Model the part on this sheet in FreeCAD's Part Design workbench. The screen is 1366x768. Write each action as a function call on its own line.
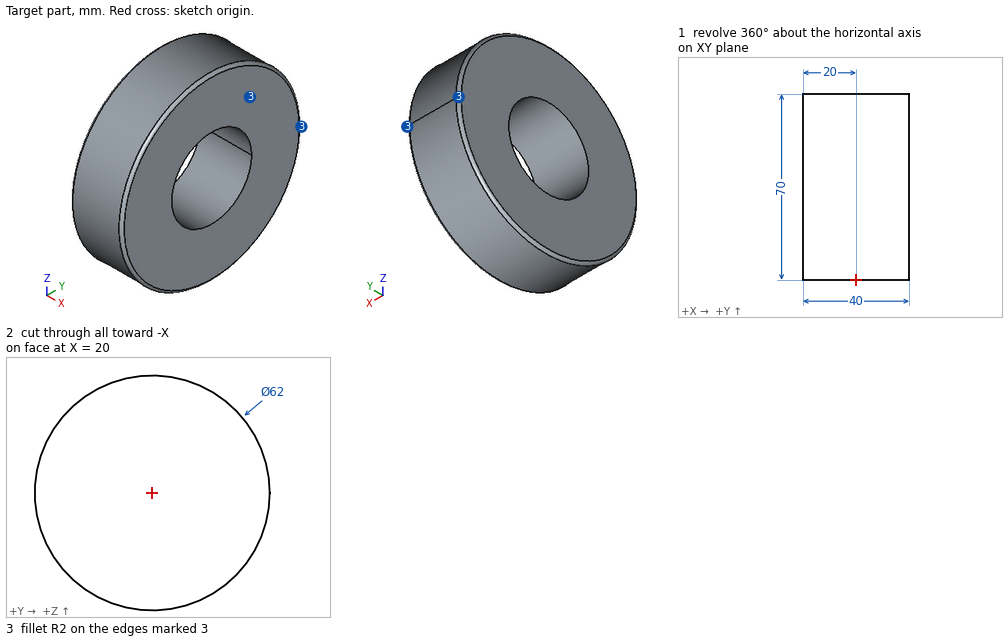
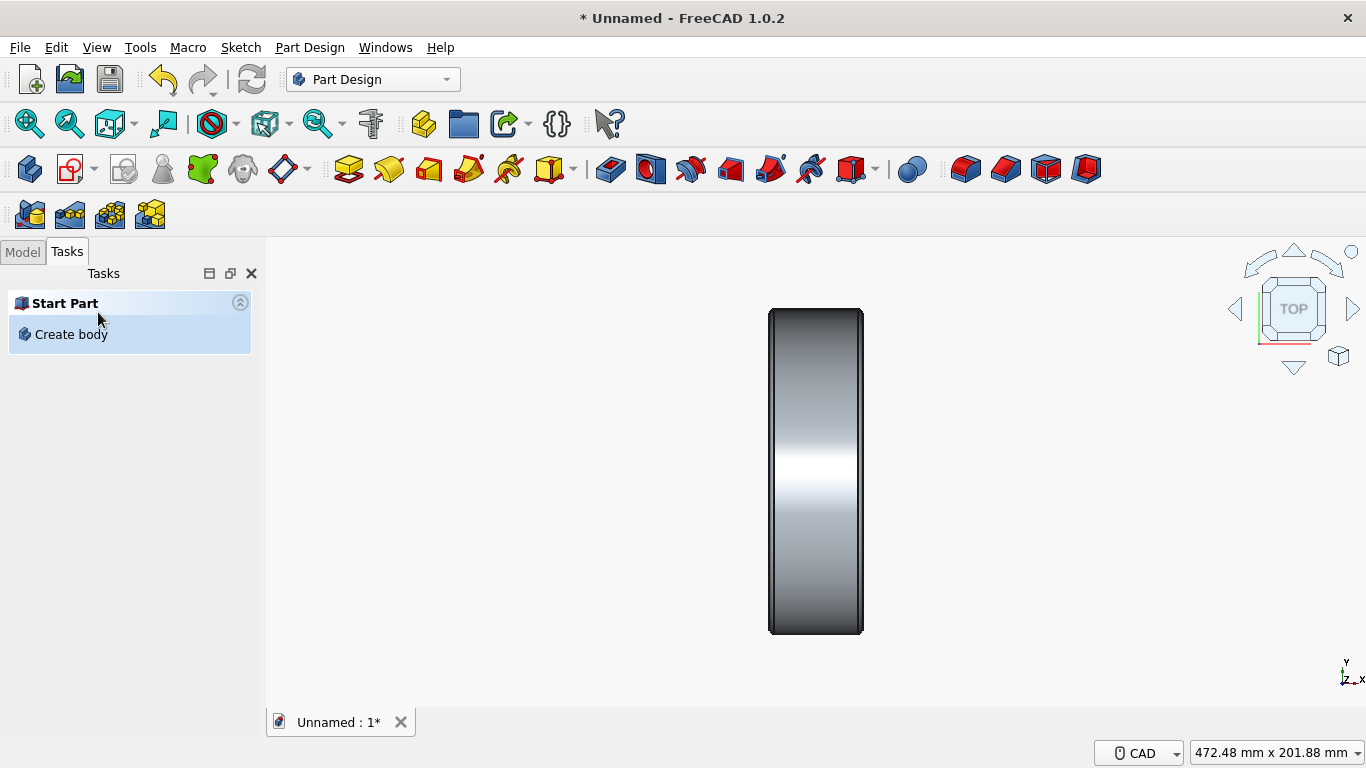
key(0)